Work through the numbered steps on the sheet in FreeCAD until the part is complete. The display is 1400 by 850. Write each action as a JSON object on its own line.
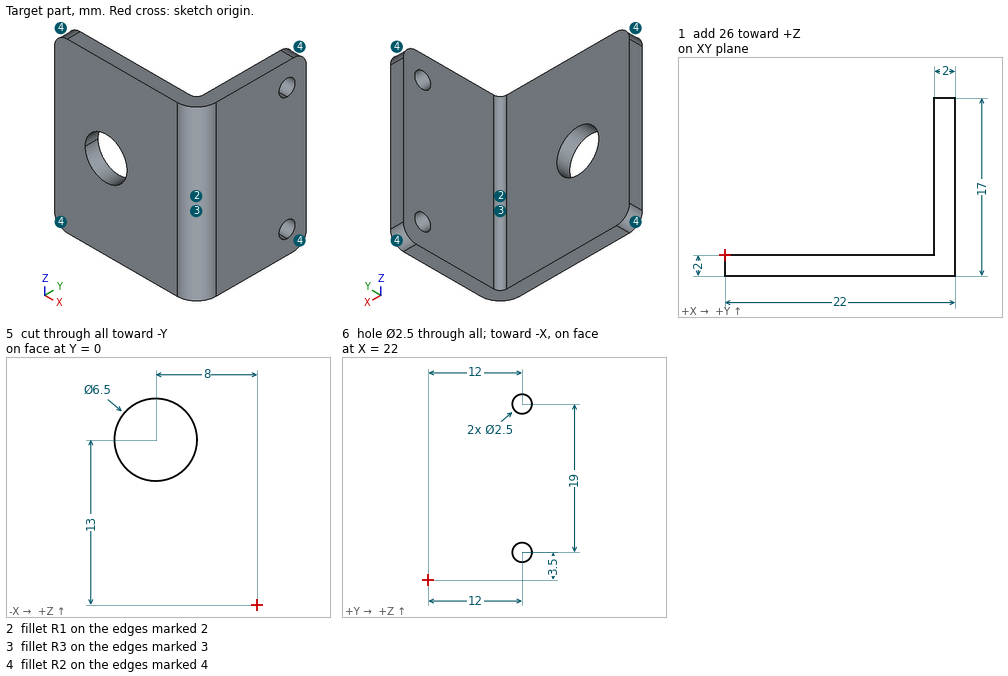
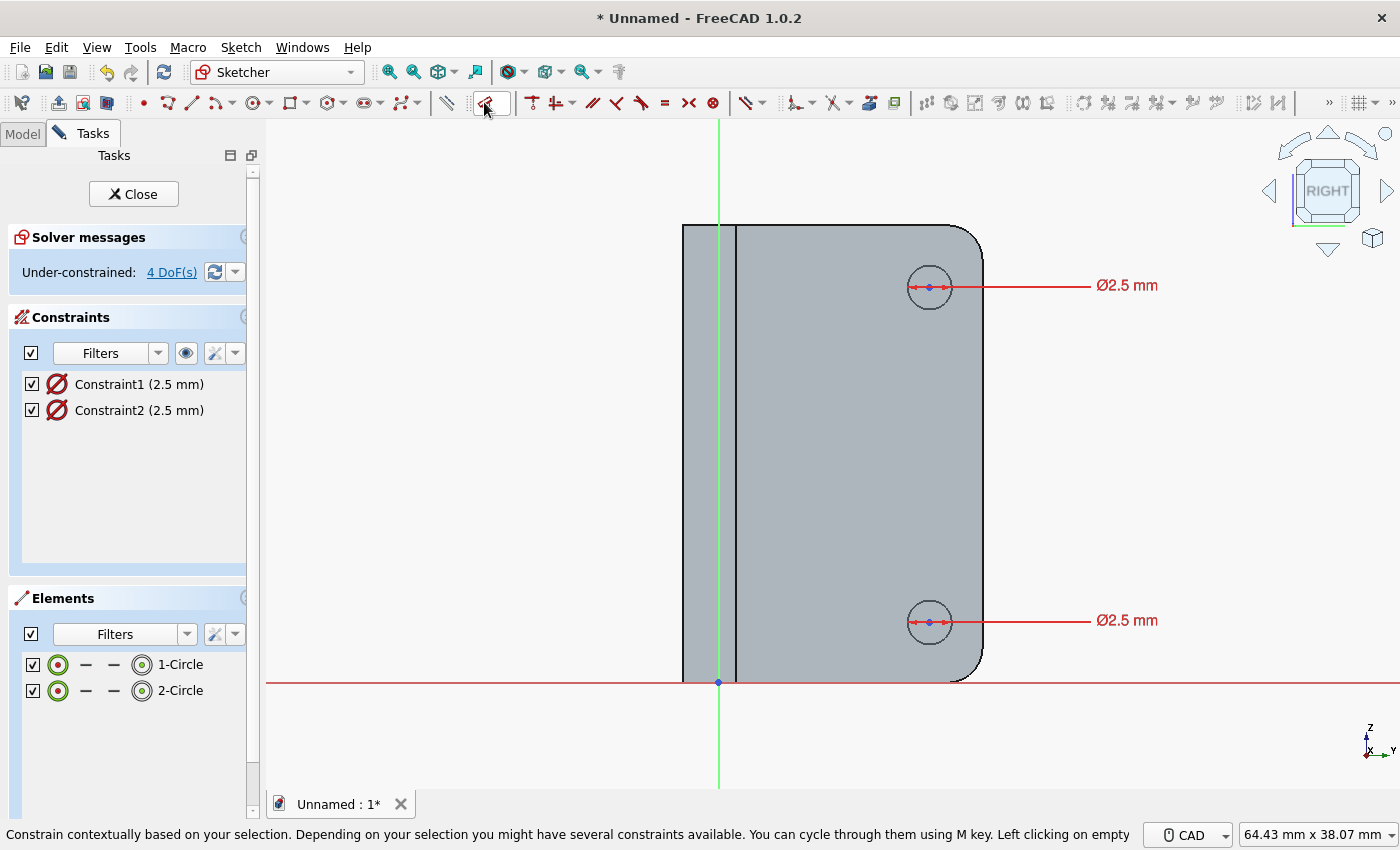
{"action": "left_click", "coordinate": [930, 287]}
{"action": "left_click", "coordinate": [824, 717]}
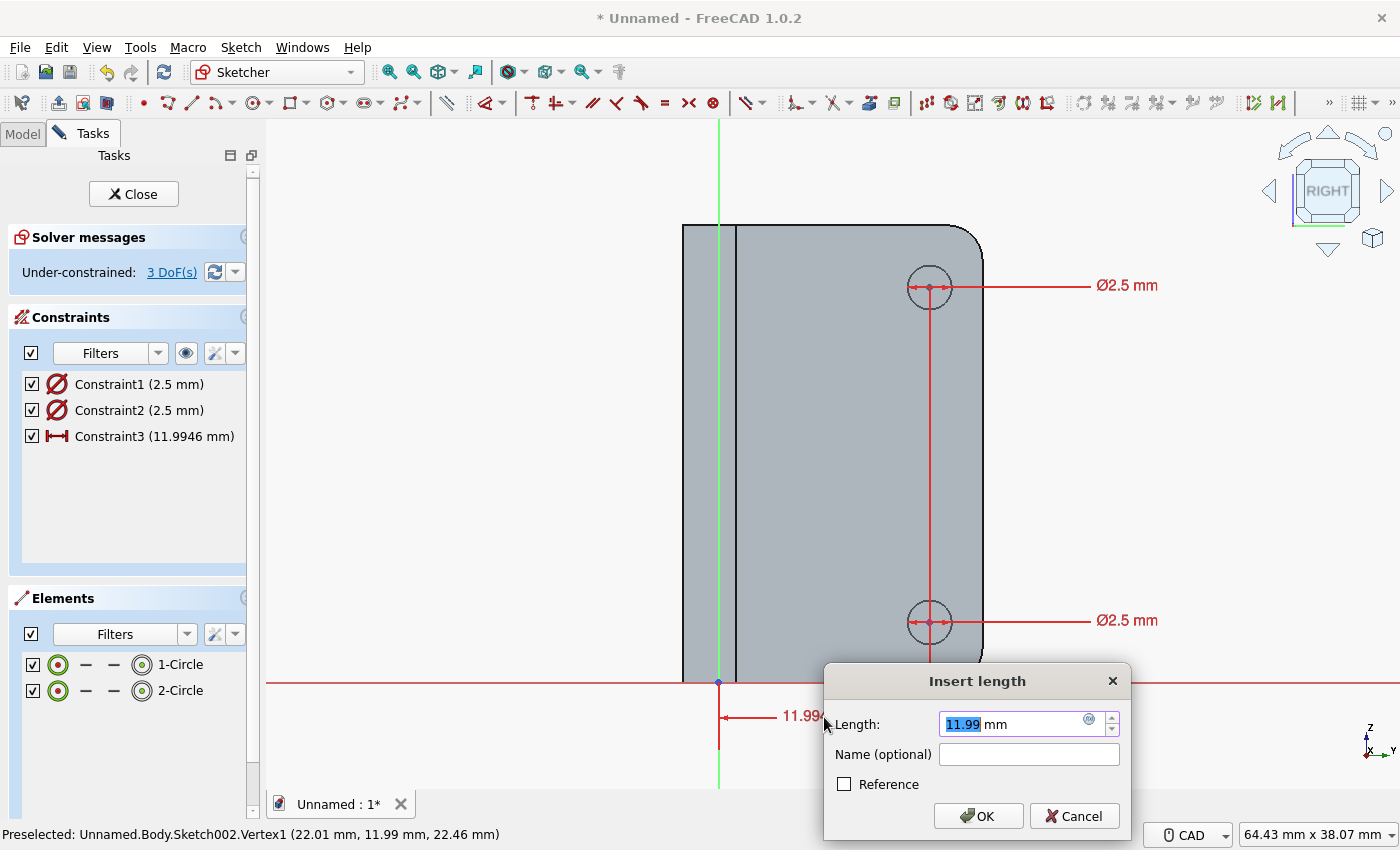
{"action": "type", "text": "12"}
{"action": "key", "text": "Return"}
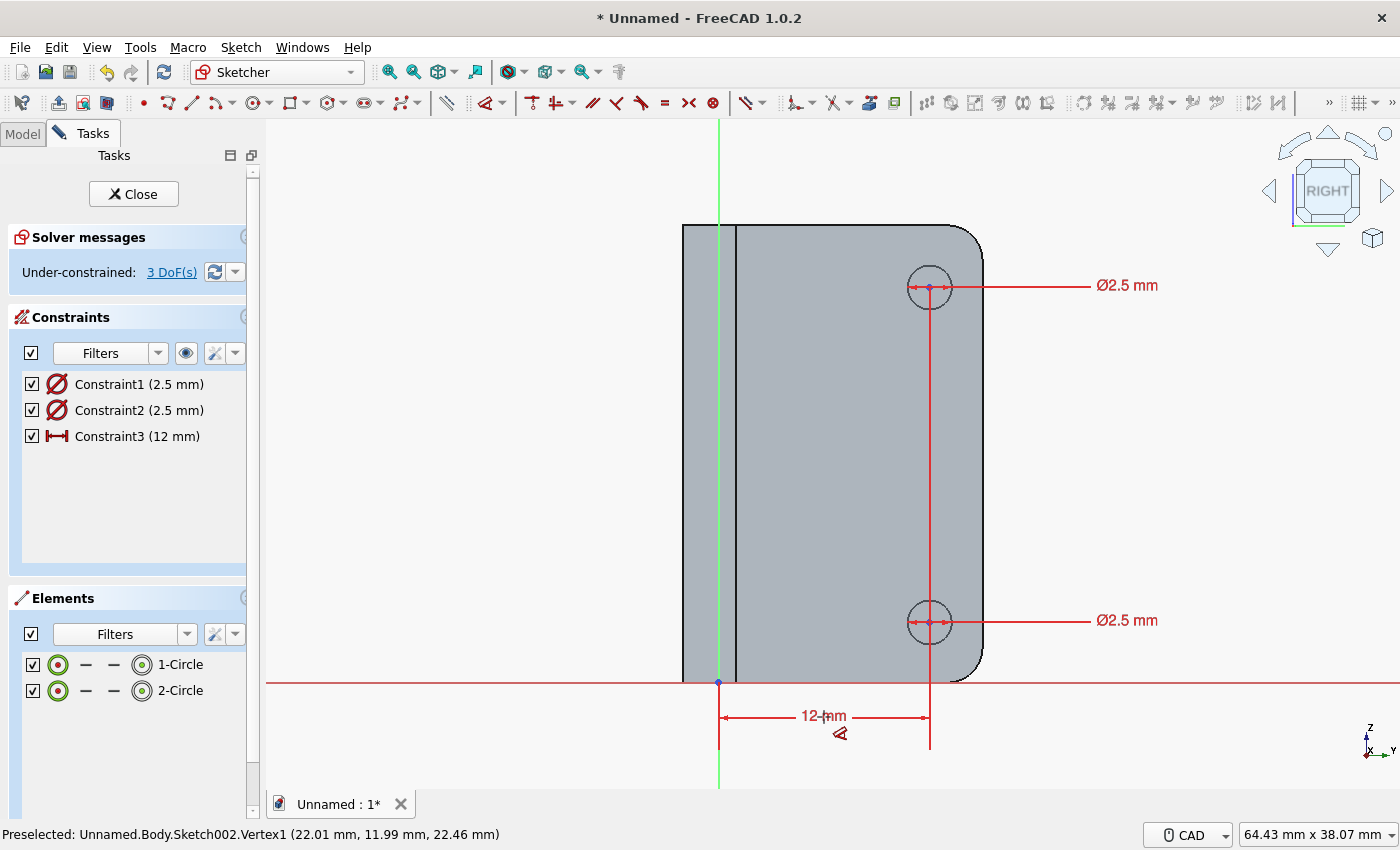
{"action": "left_click", "coordinate": [930, 622]}
{"action": "left_click", "coordinate": [750, 717]}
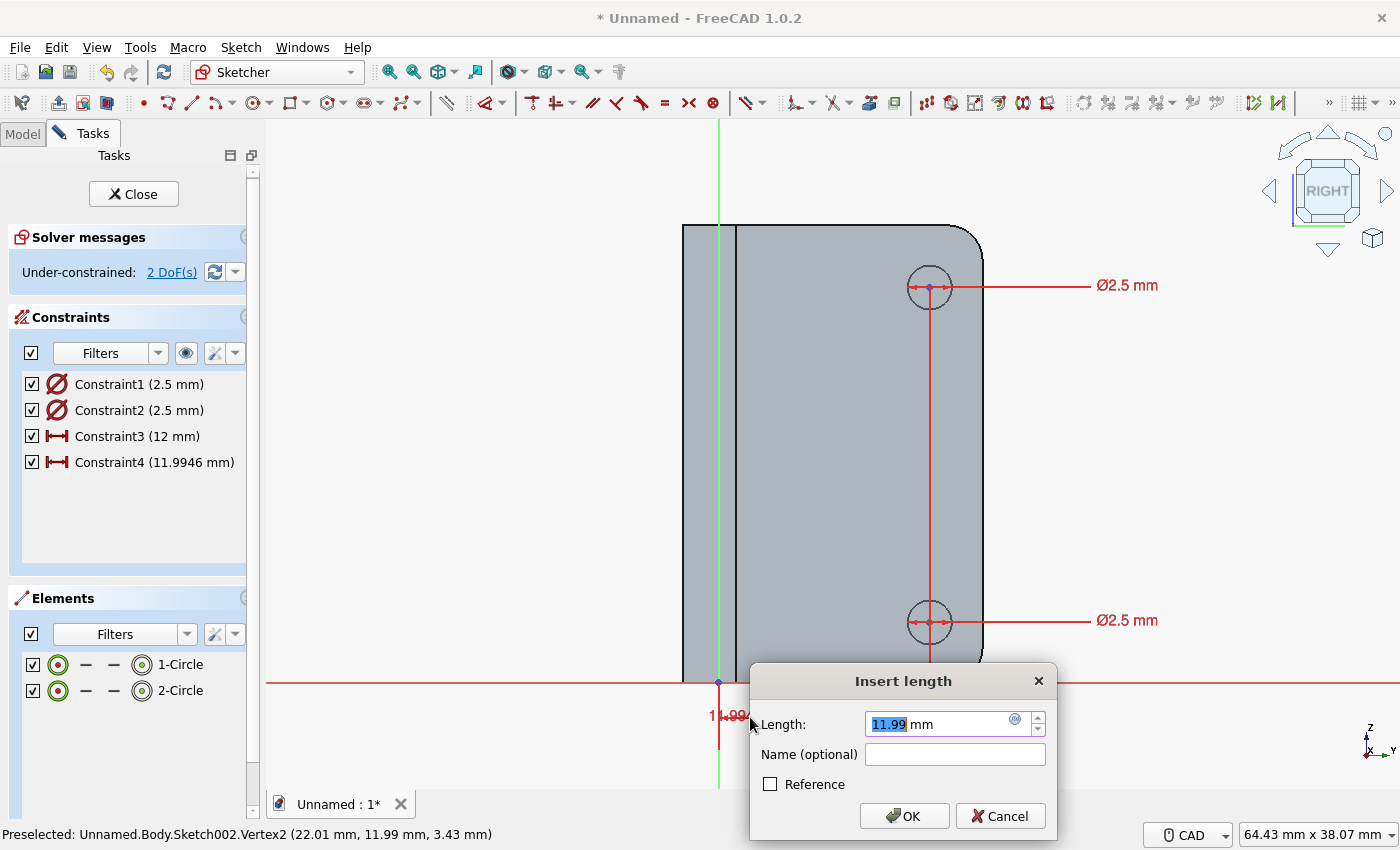
{"action": "type", "text": "12"}
{"action": "key", "text": "Return"}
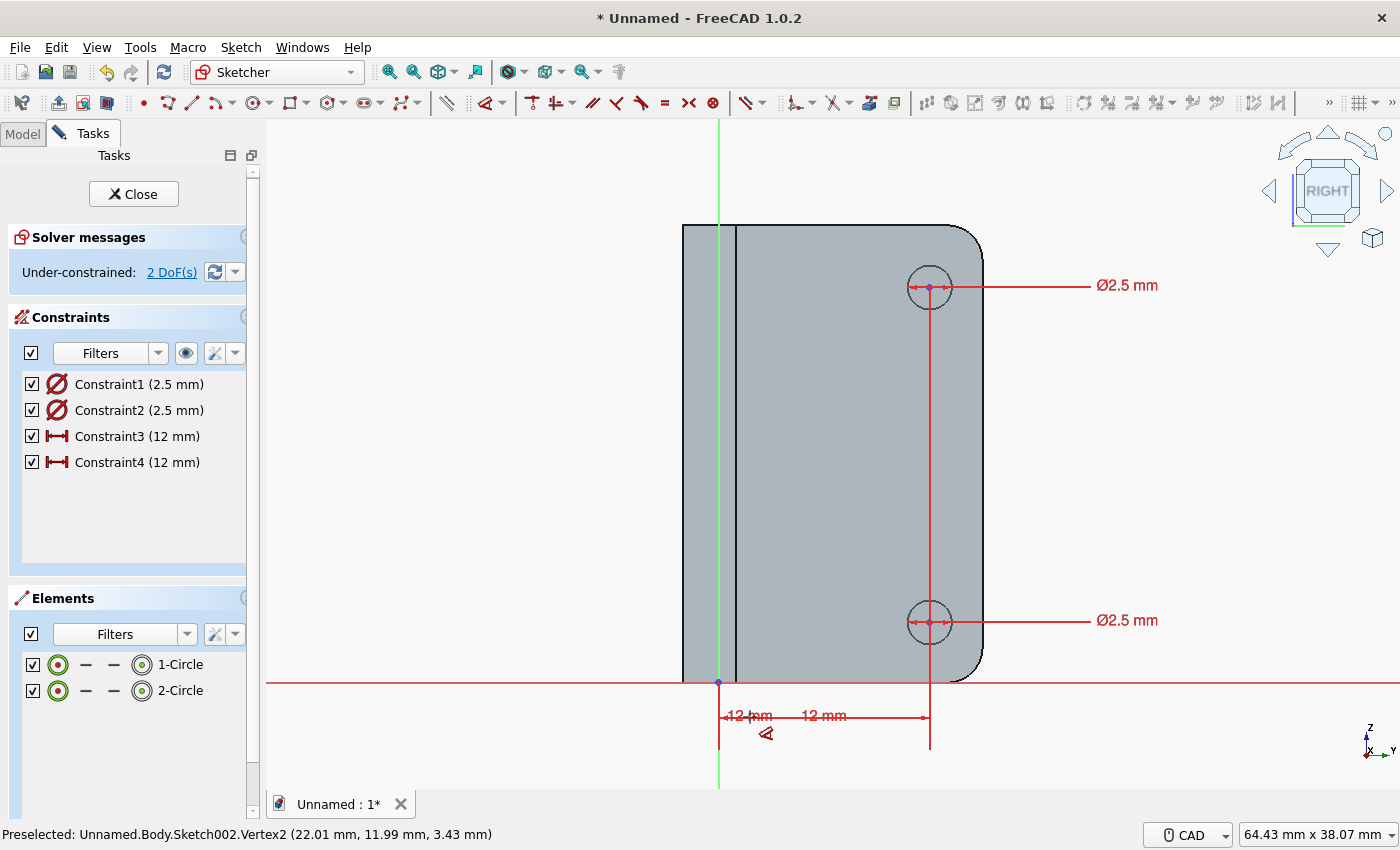
{"action": "left_click", "coordinate": [930, 622]}
{"action": "left_click", "coordinate": [685, 653]}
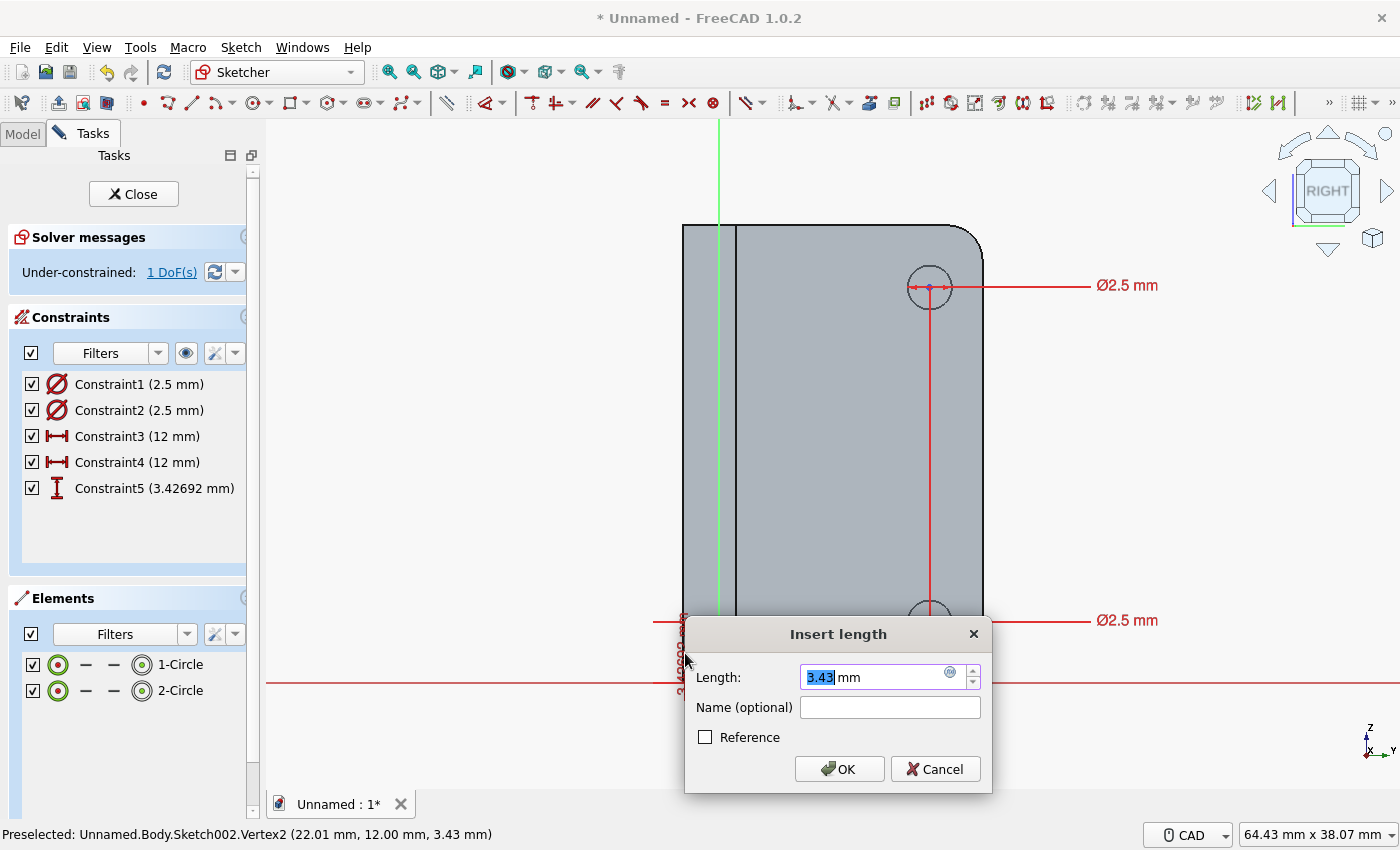
{"action": "type", "text": "3.5"}
{"action": "key", "text": "Return"}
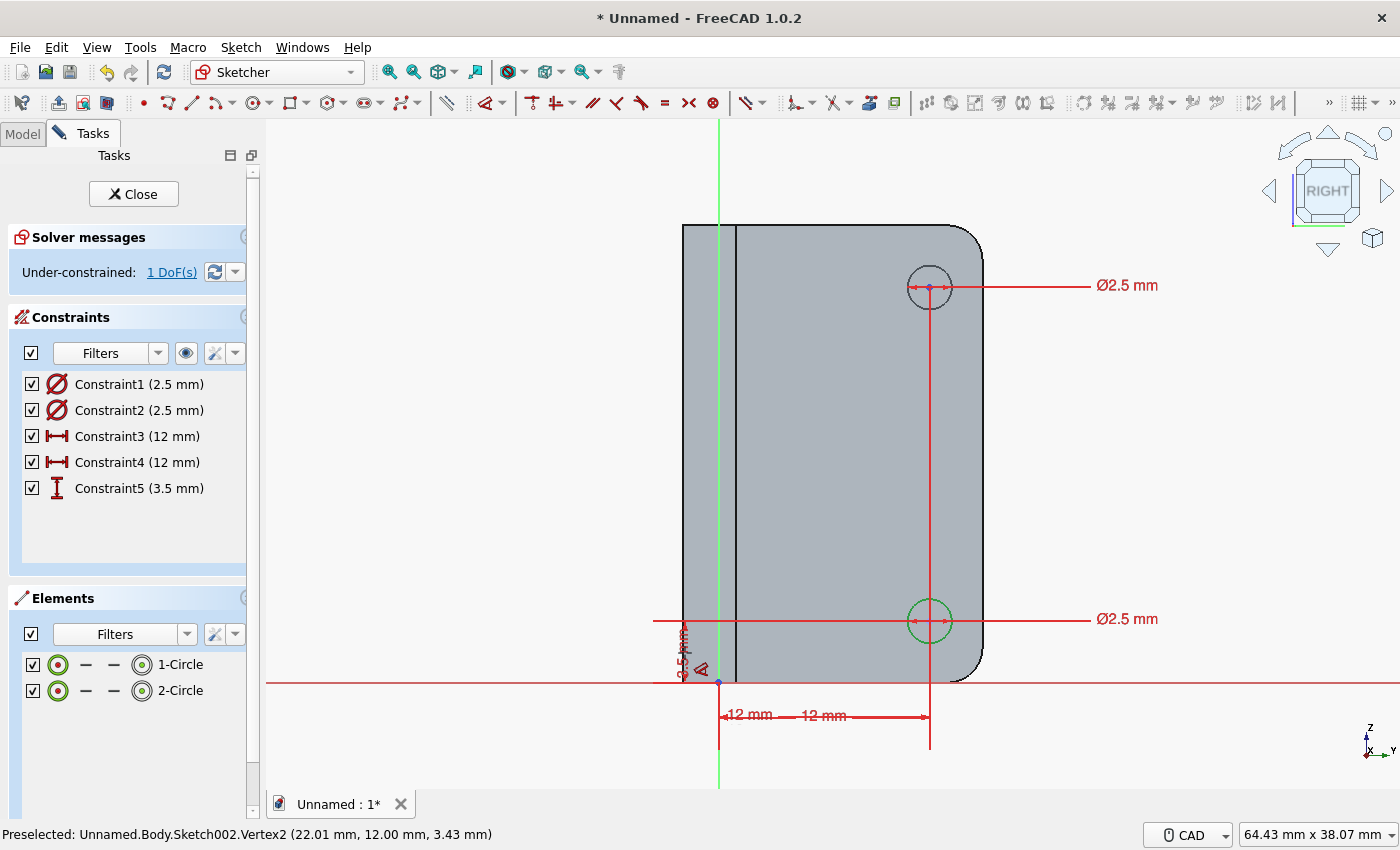
{"action": "left_click", "coordinate": [930, 287]}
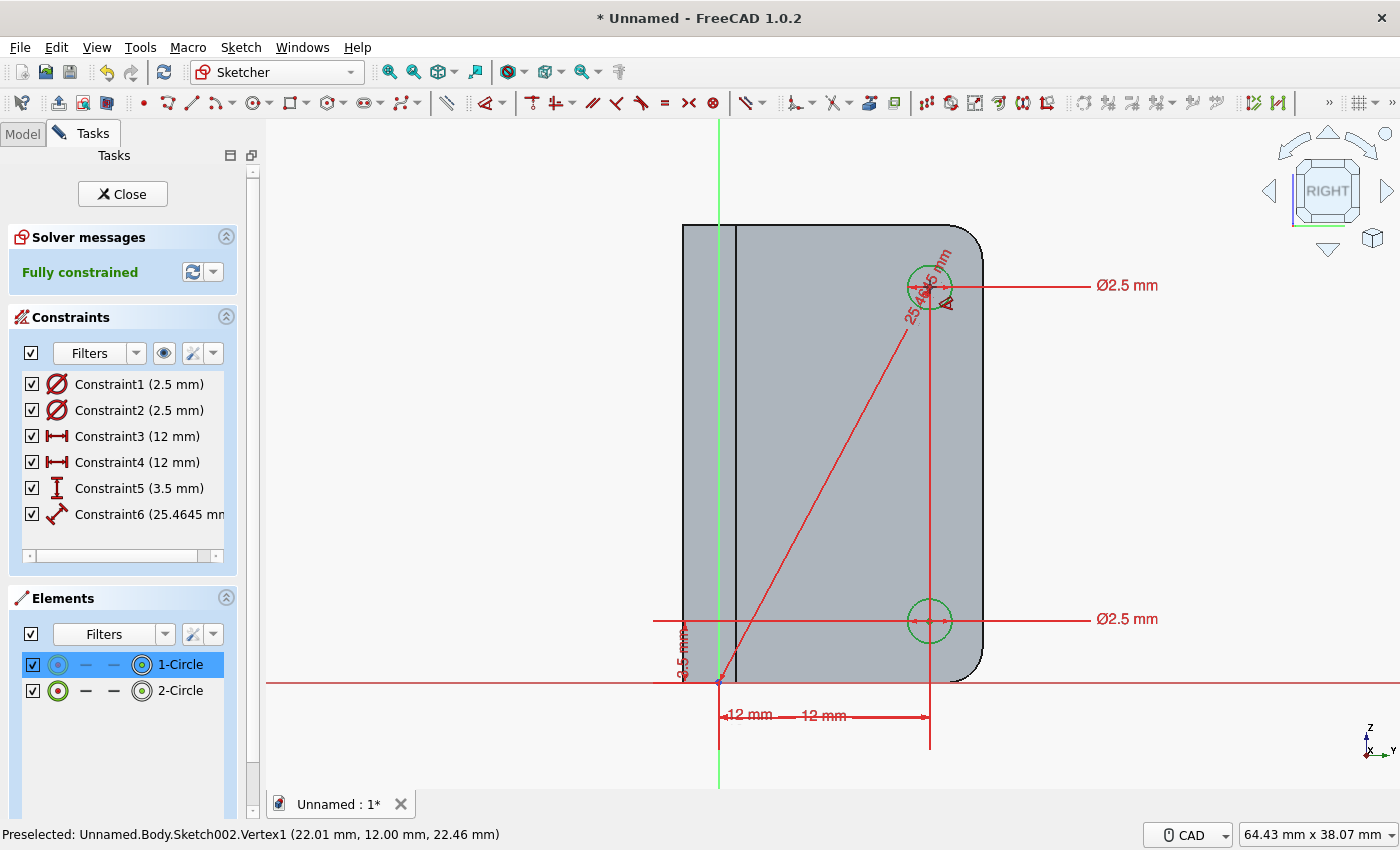
{"action": "left_click", "coordinate": [930, 621]}
{"action": "left_click", "coordinate": [964, 454]}